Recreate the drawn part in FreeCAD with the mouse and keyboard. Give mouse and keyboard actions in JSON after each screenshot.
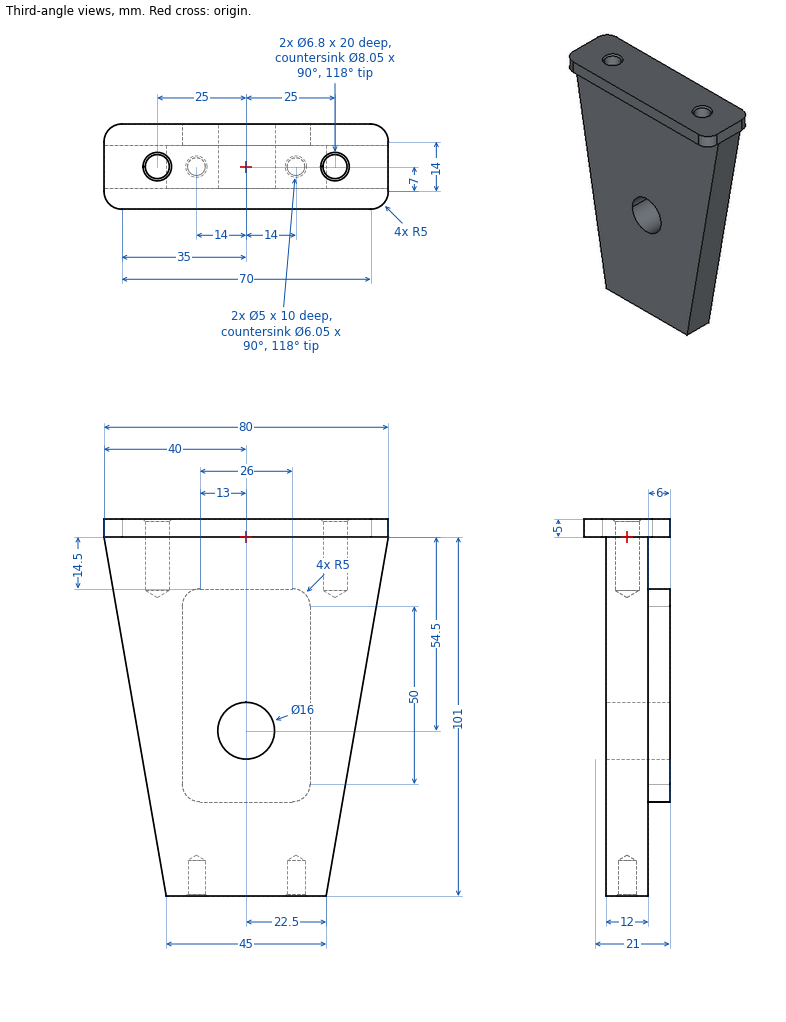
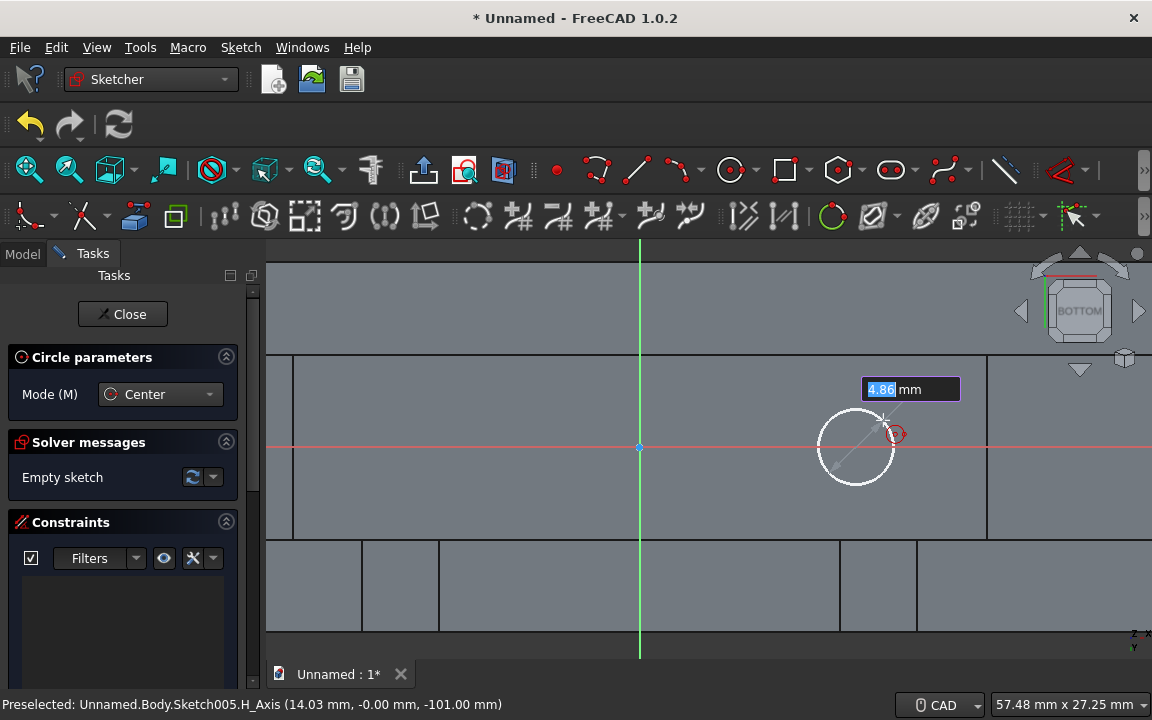
{"action": "type", "text": "5"}
{"action": "key", "text": "Return"}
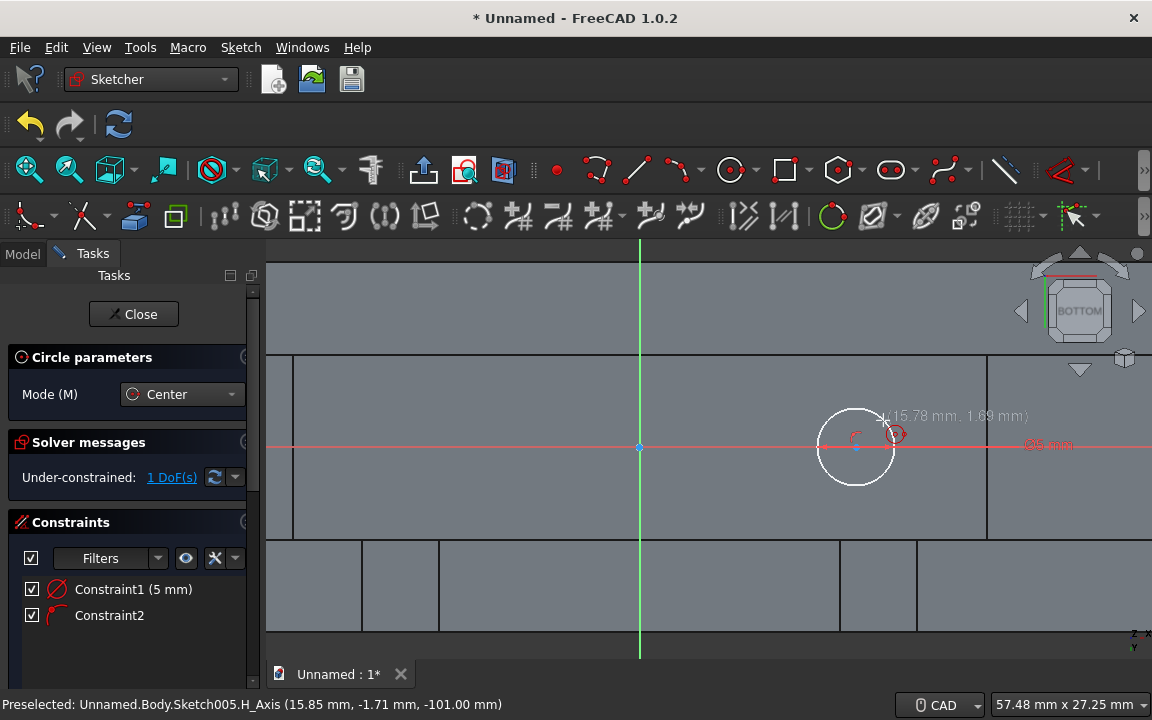
{"action": "left_click", "coordinate": [424, 447]}
{"action": "mouse_move", "coordinate": [451, 420]}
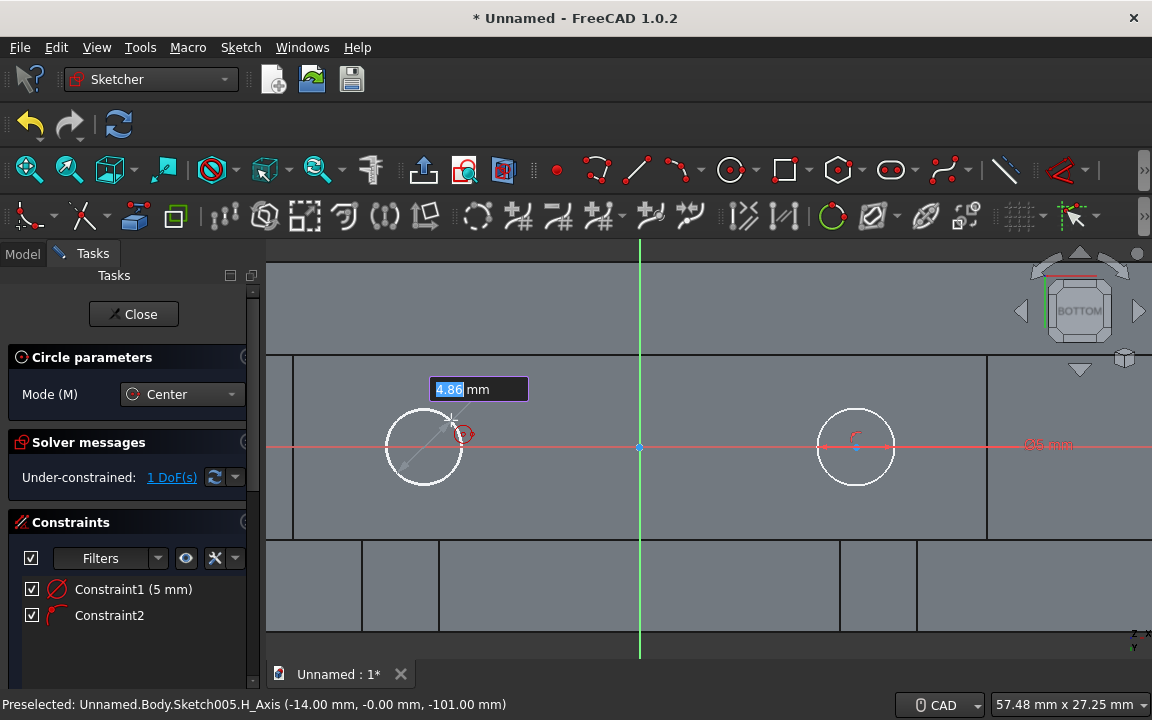
{"action": "type", "text": "5"}
{"action": "key", "text": "Return"}
{"action": "key", "text": "Escape"}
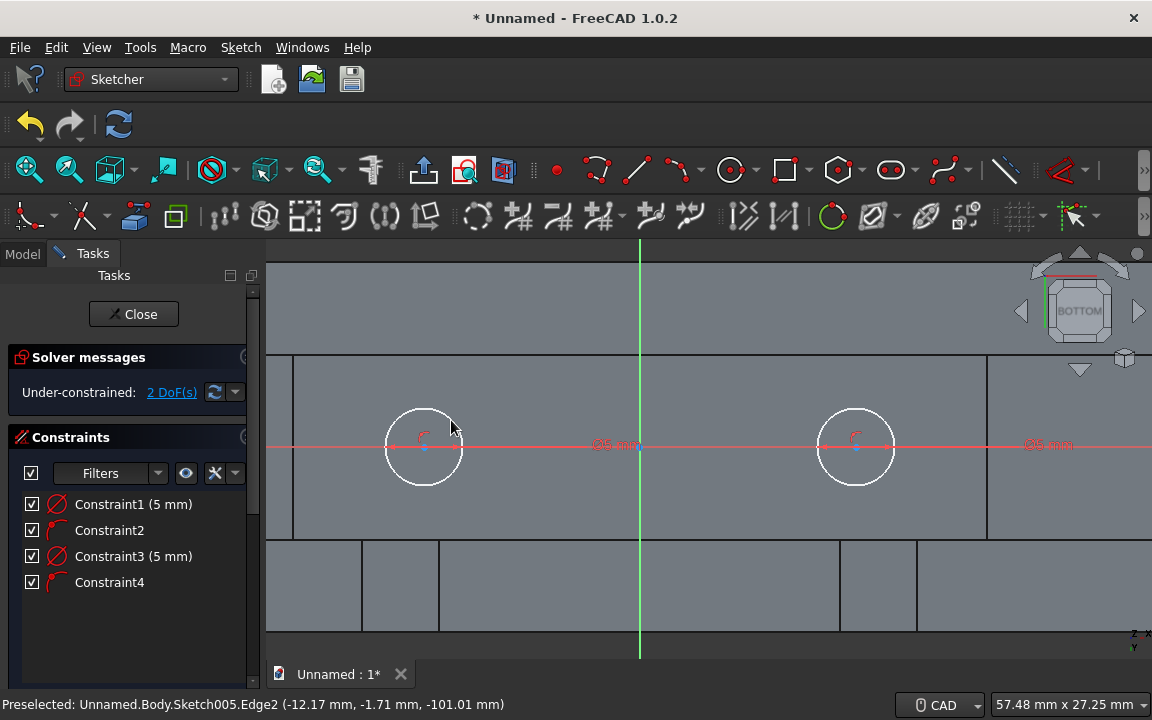
{"action": "left_click", "coordinate": [1060, 170]}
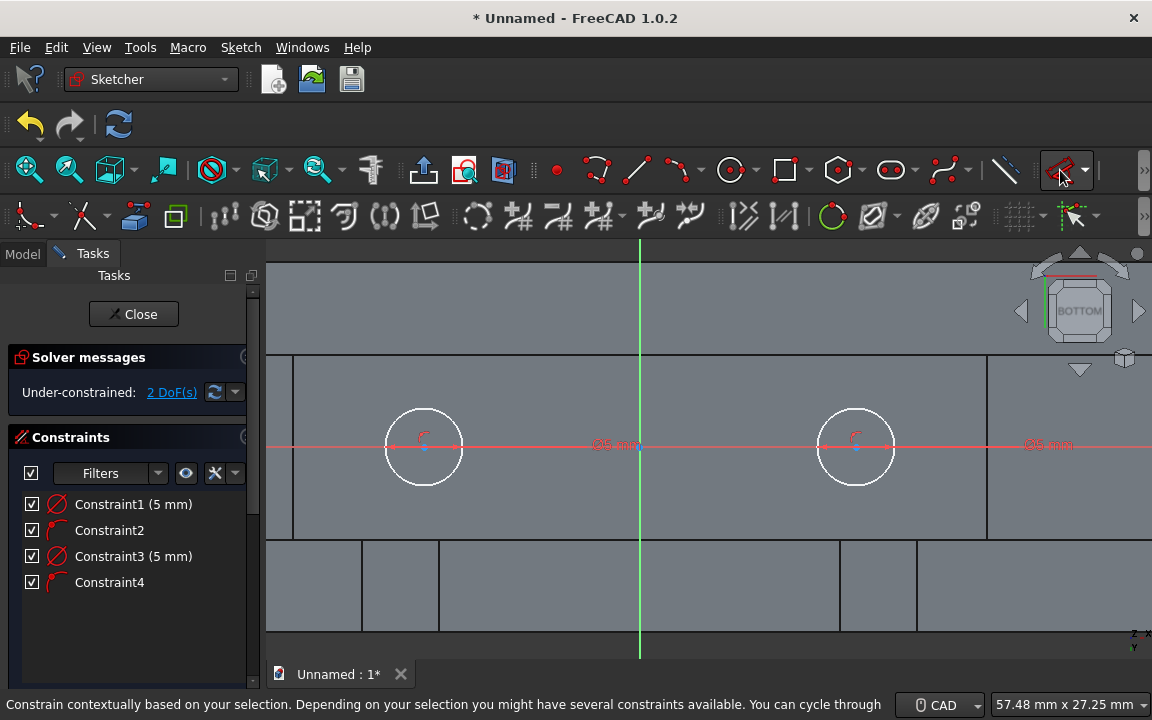
{"action": "left_click", "coordinate": [856, 447]}
{"action": "left_click", "coordinate": [748, 481]}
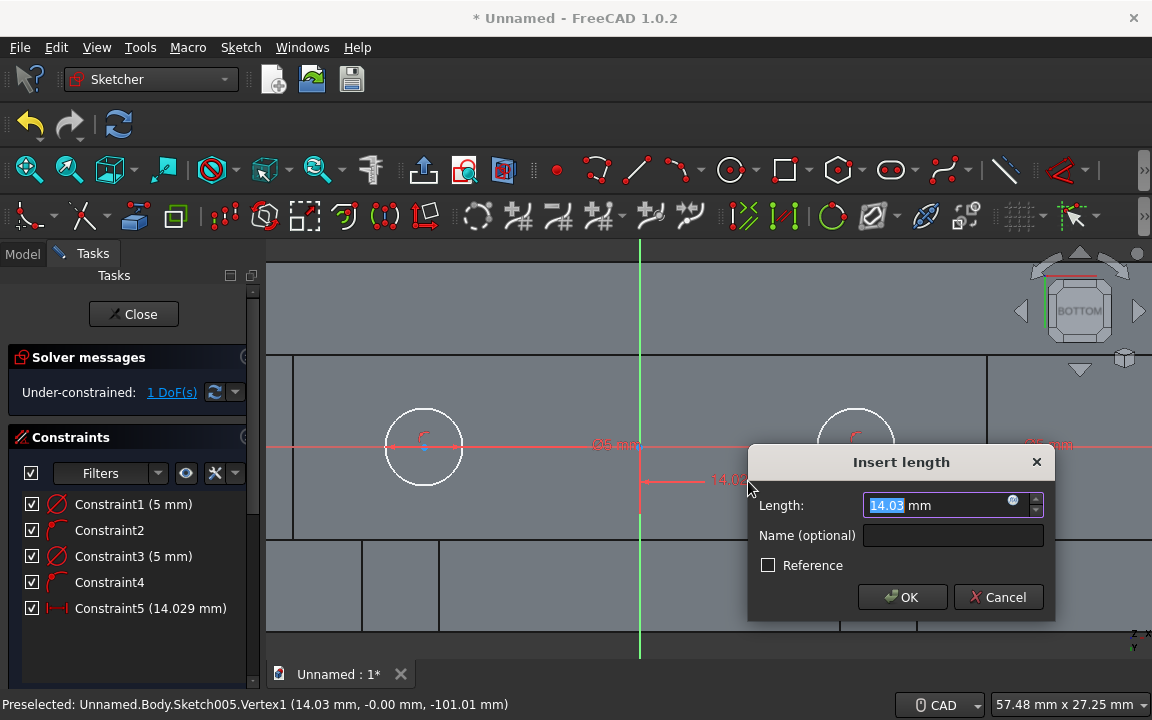
{"action": "type", "text": "14"}
{"action": "key", "text": "Return"}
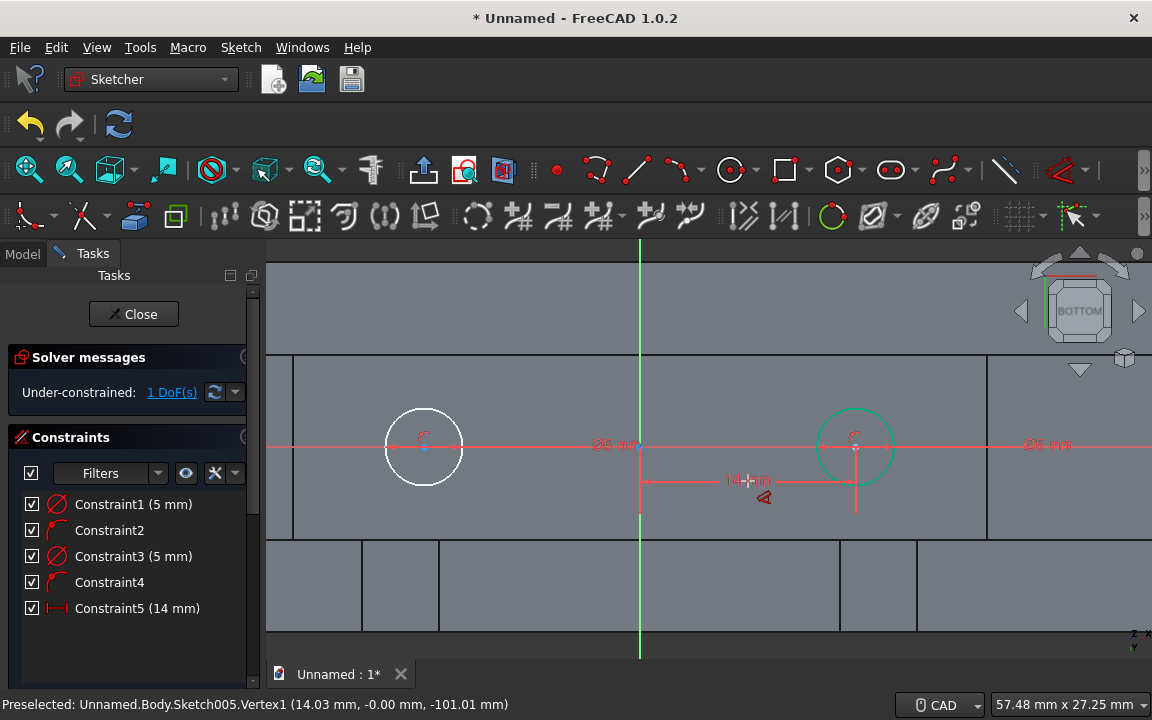
{"action": "left_click", "coordinate": [424, 447]}
{"action": "left_click", "coordinate": [532, 481]}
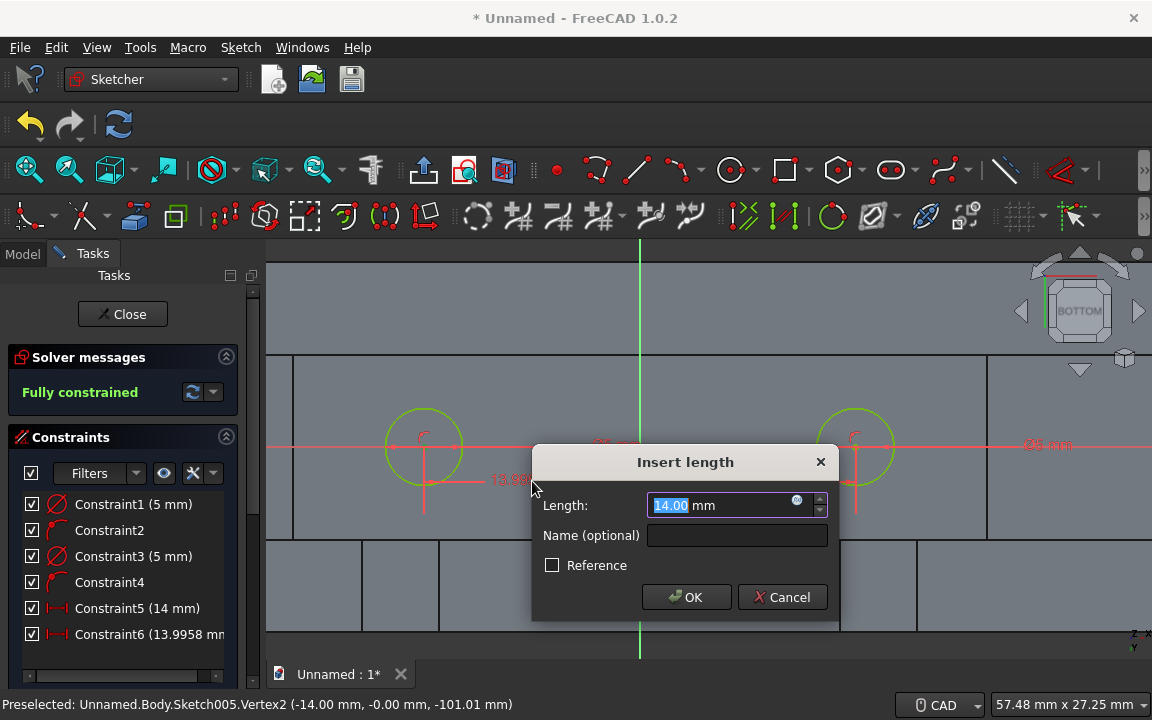
{"action": "type", "text": "14"}
{"action": "key", "text": "Return"}
{"action": "key", "text": "Escape"}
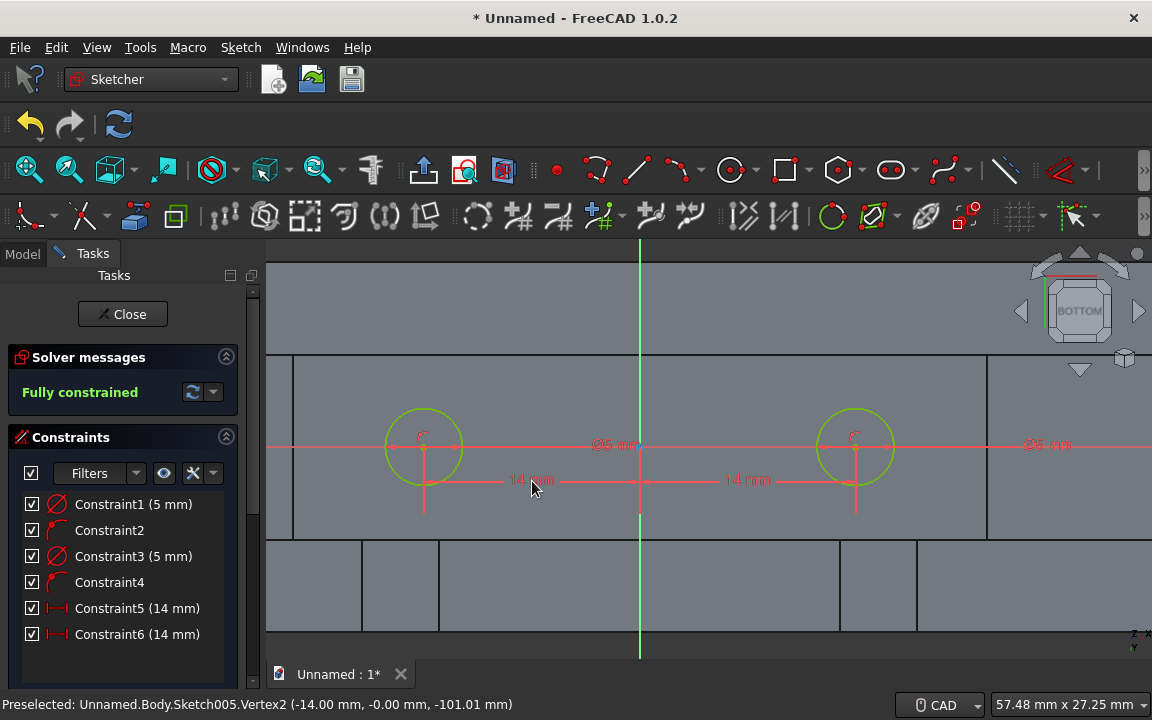
{"action": "left_click", "coordinate": [123, 314]}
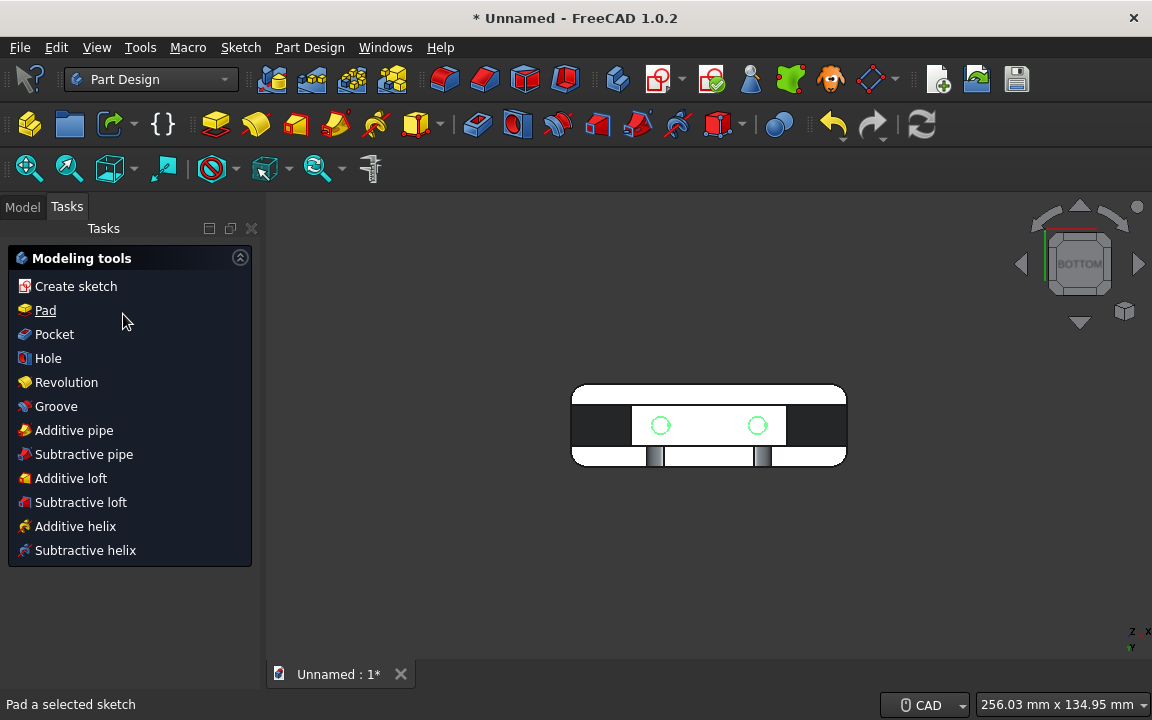
{"action": "left_click", "coordinate": [518, 124]}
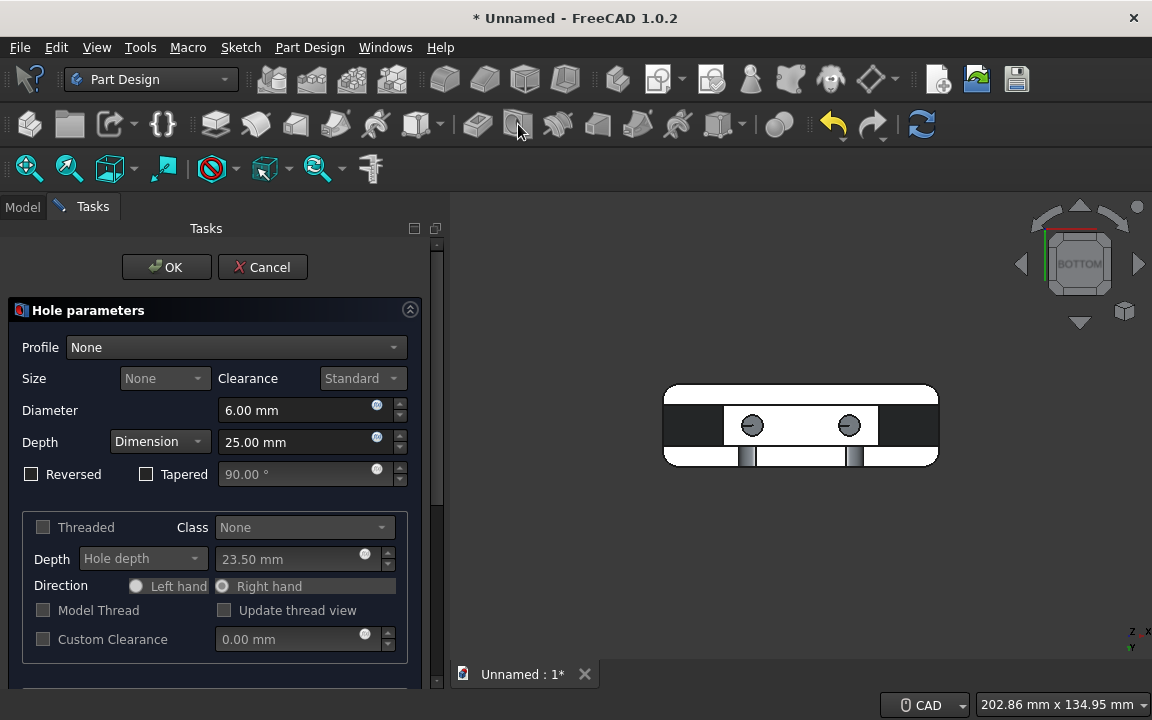
{"action": "triple_click", "coordinate": [305, 410]}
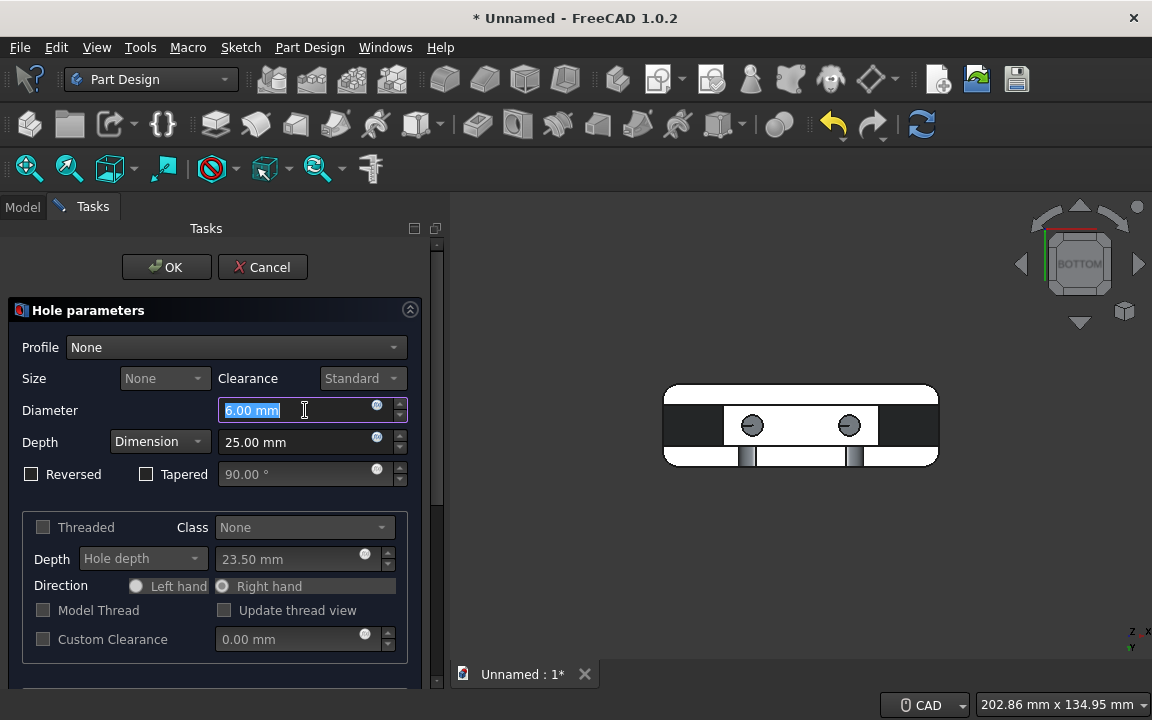
{"action": "type", "text": "5"}
{"action": "key", "text": "Tab"}